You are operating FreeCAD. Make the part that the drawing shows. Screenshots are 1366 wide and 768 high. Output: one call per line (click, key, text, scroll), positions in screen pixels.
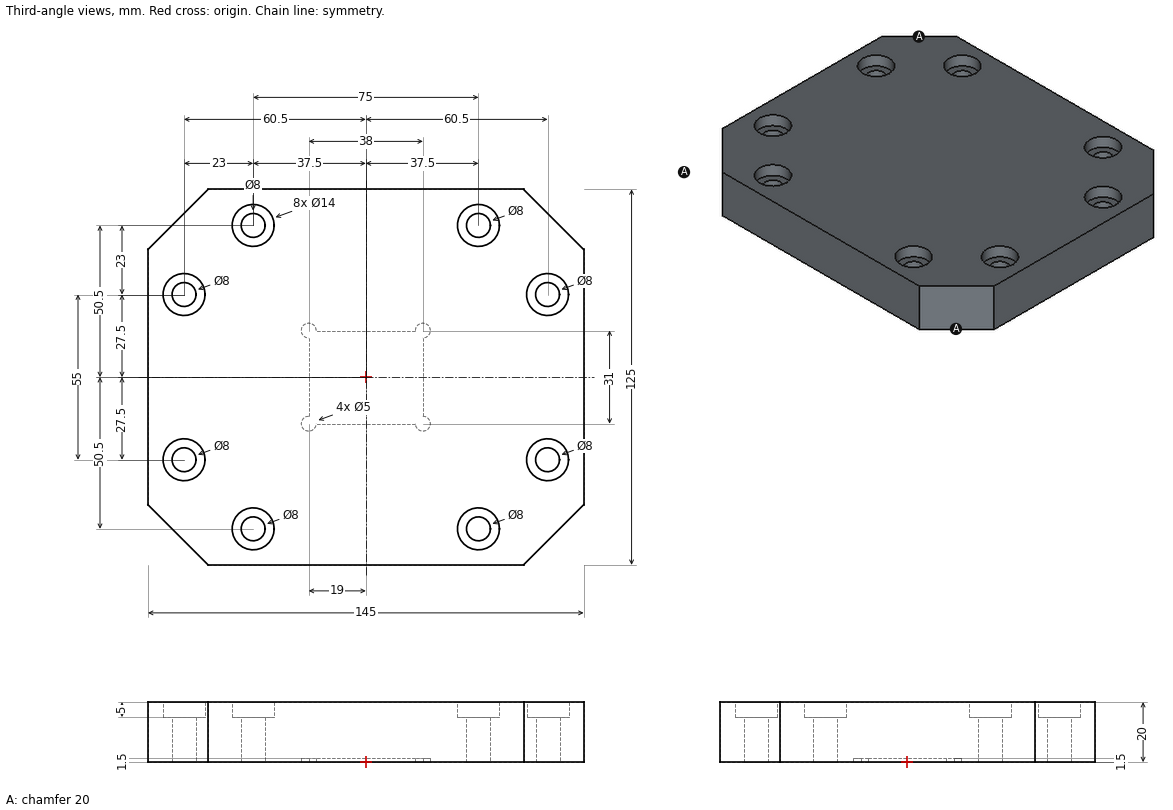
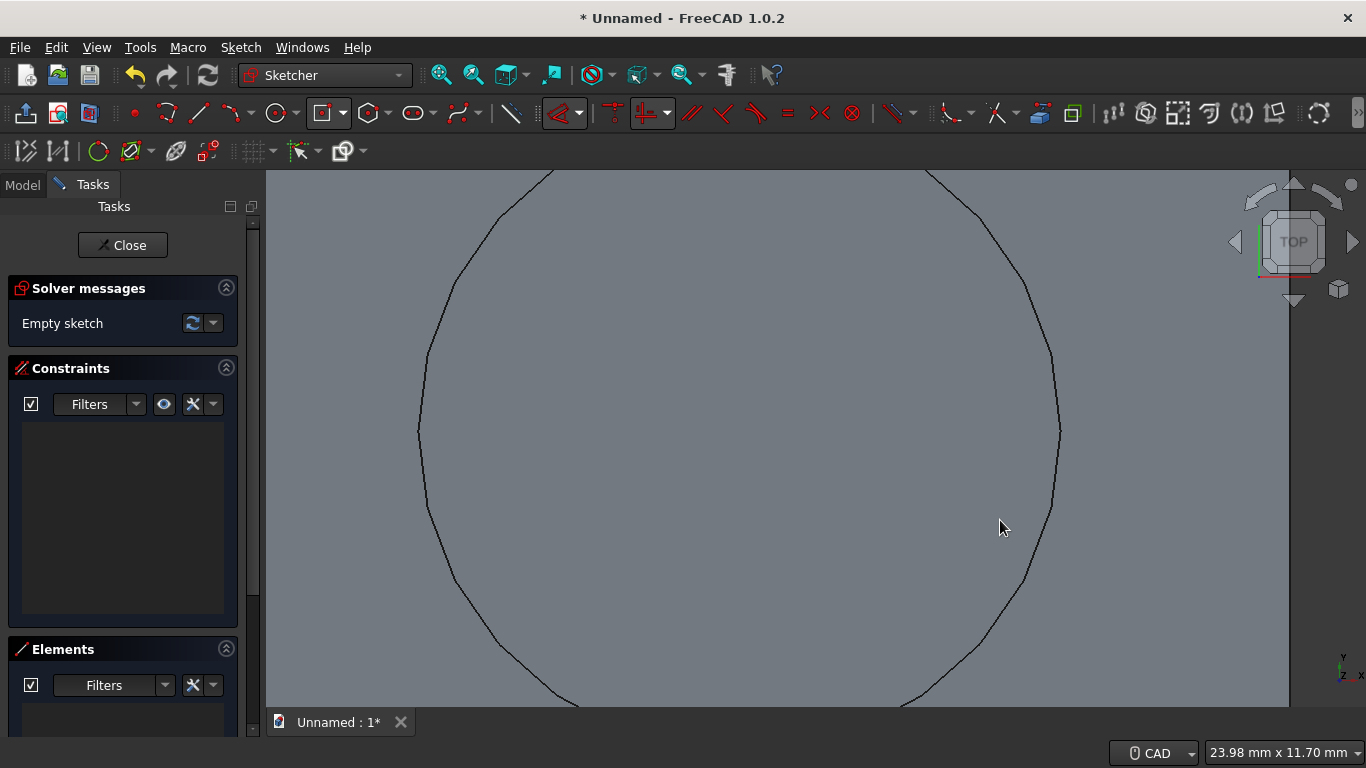
key(g)
key(c)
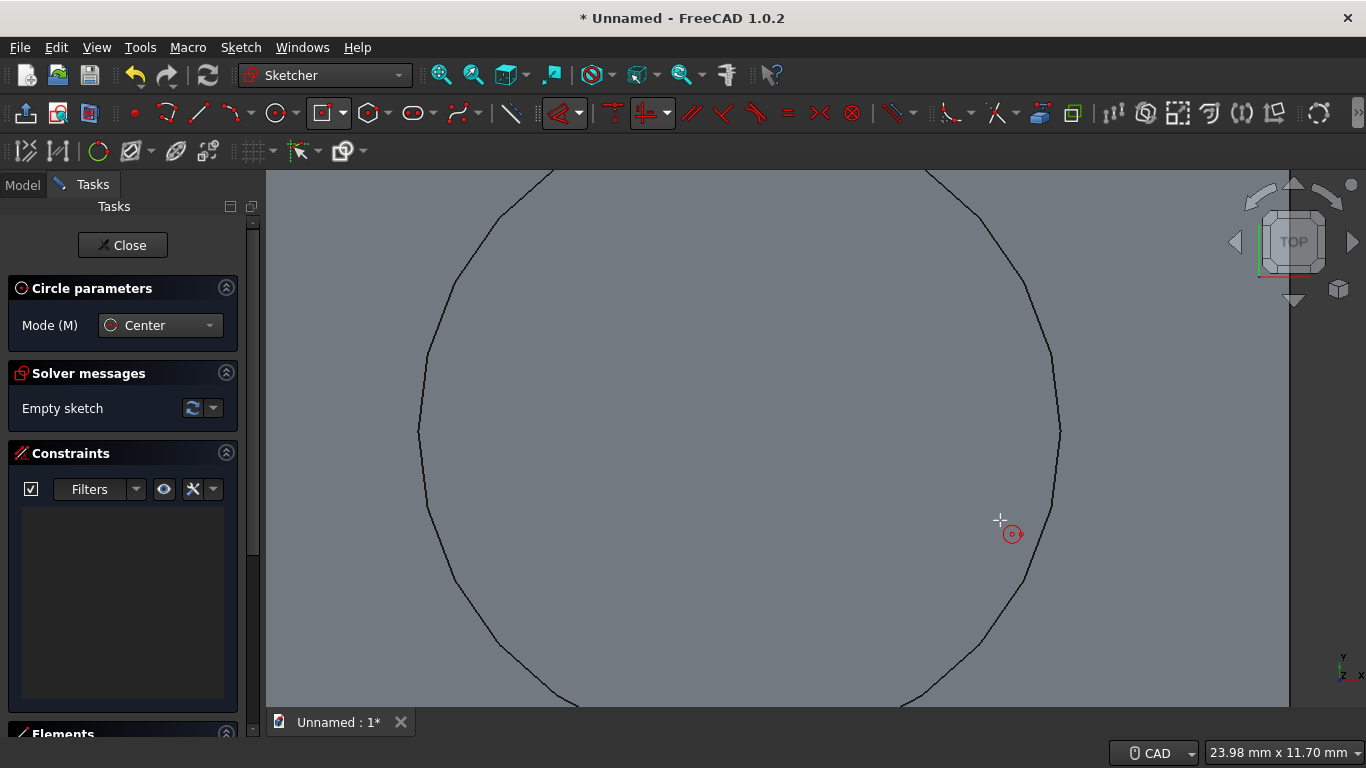
click(739, 431)
click(869, 302)
key(Escape)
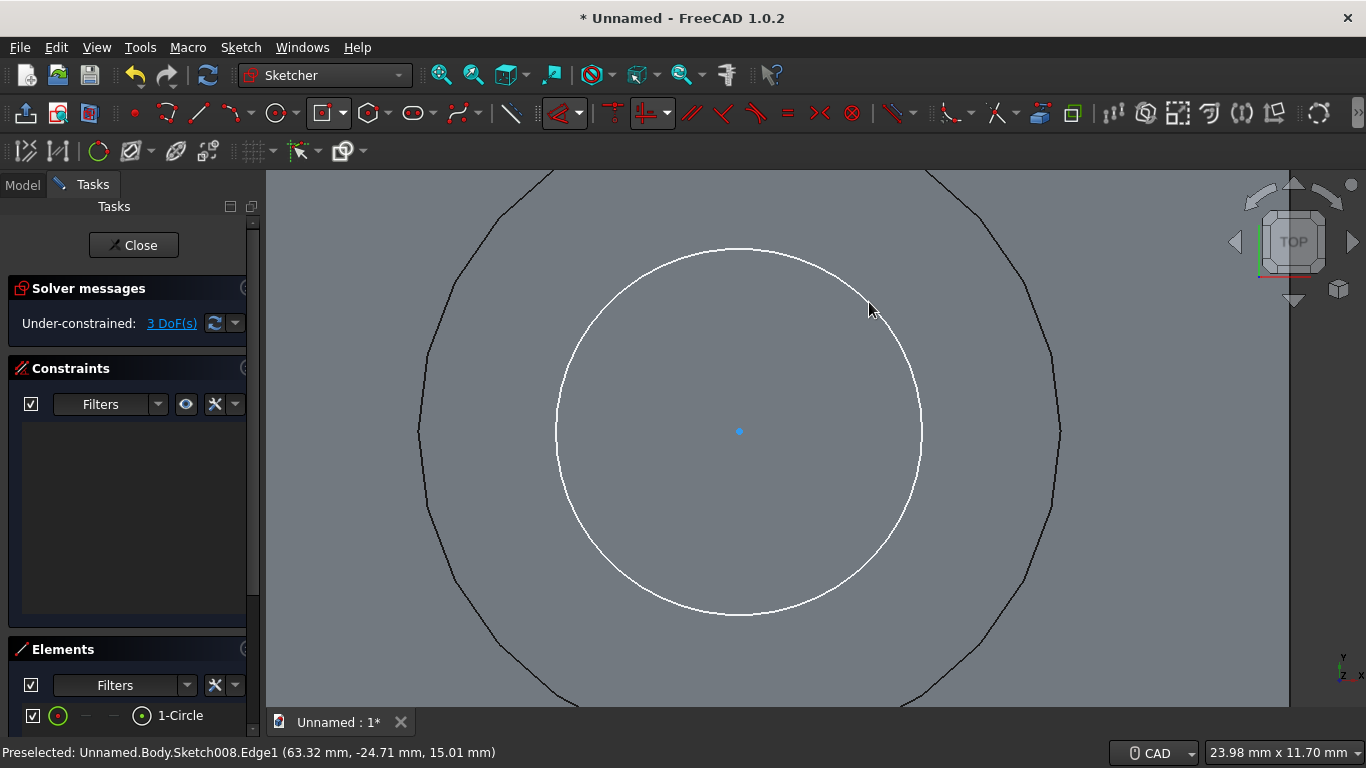
click(868, 302)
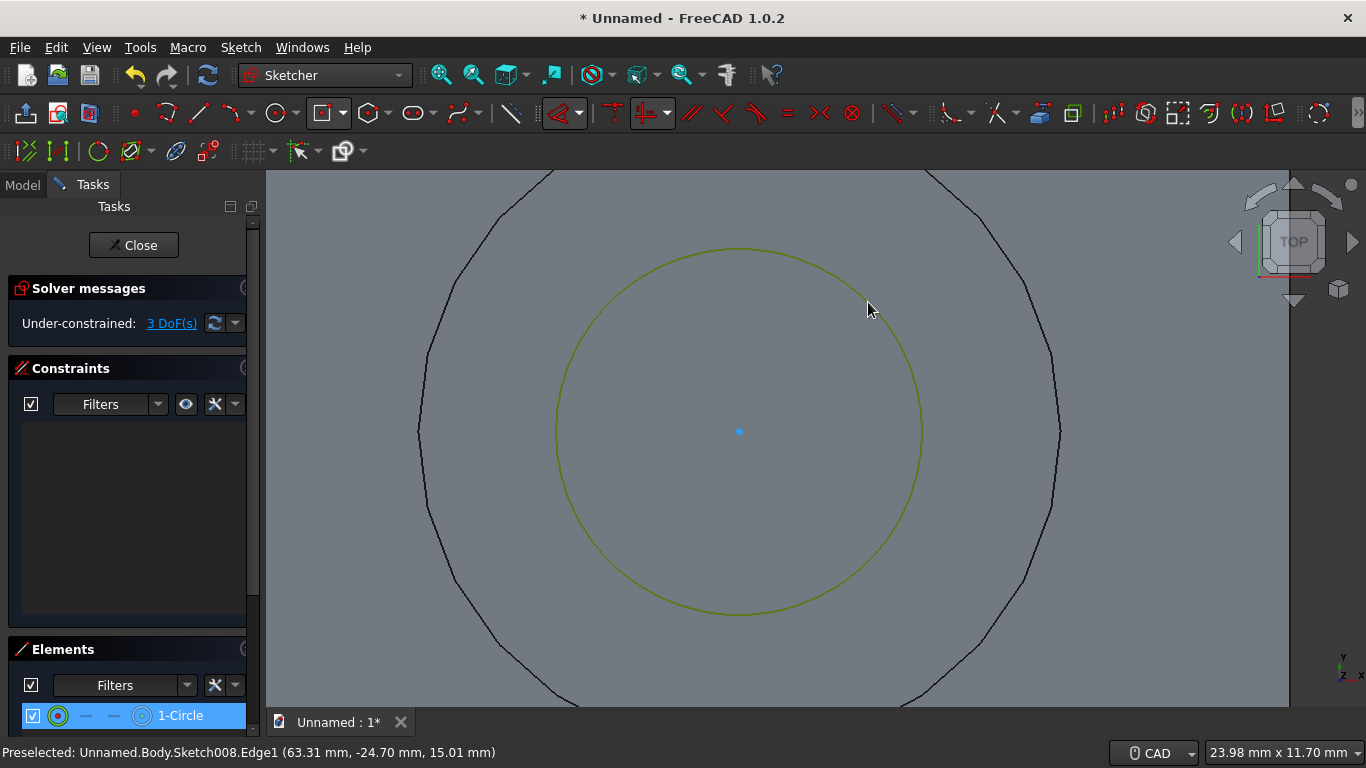
key(k)
key(o)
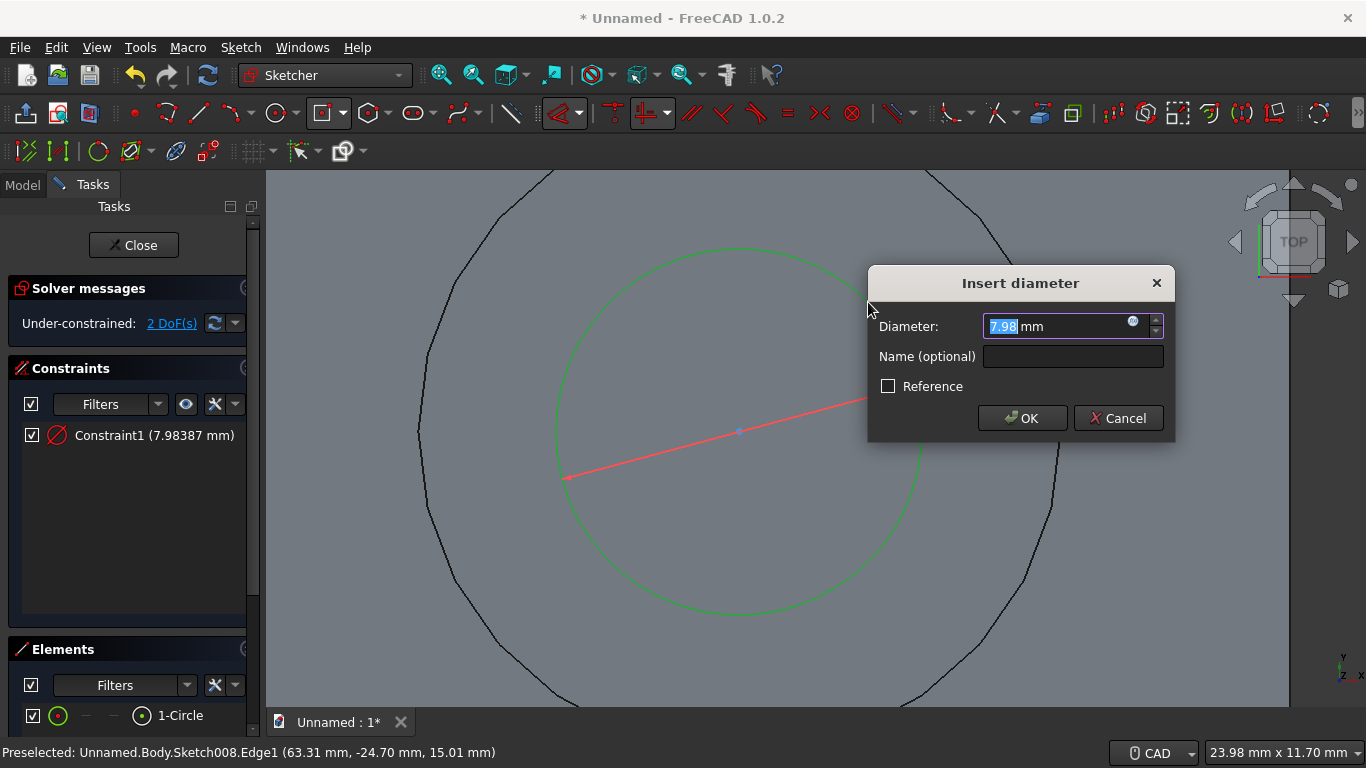
text(8)
key(Return)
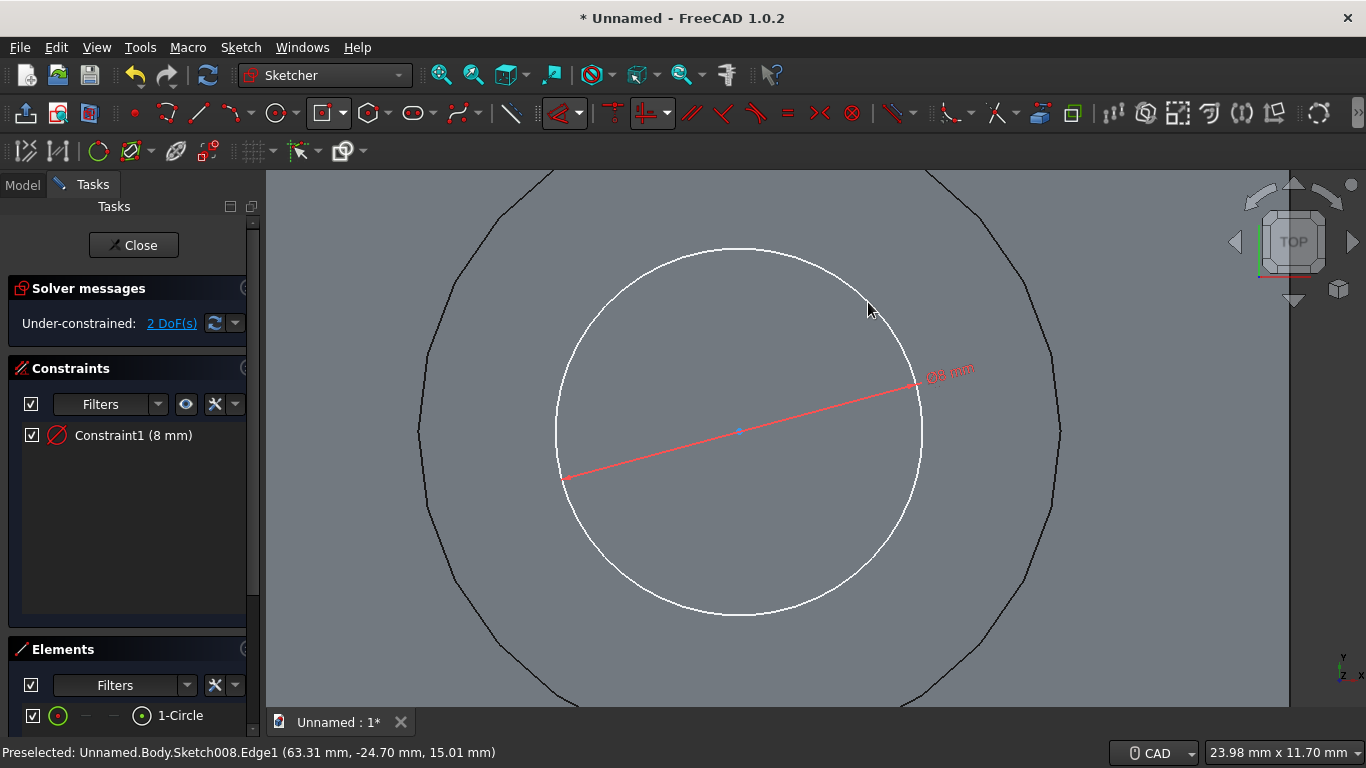
click(739, 432)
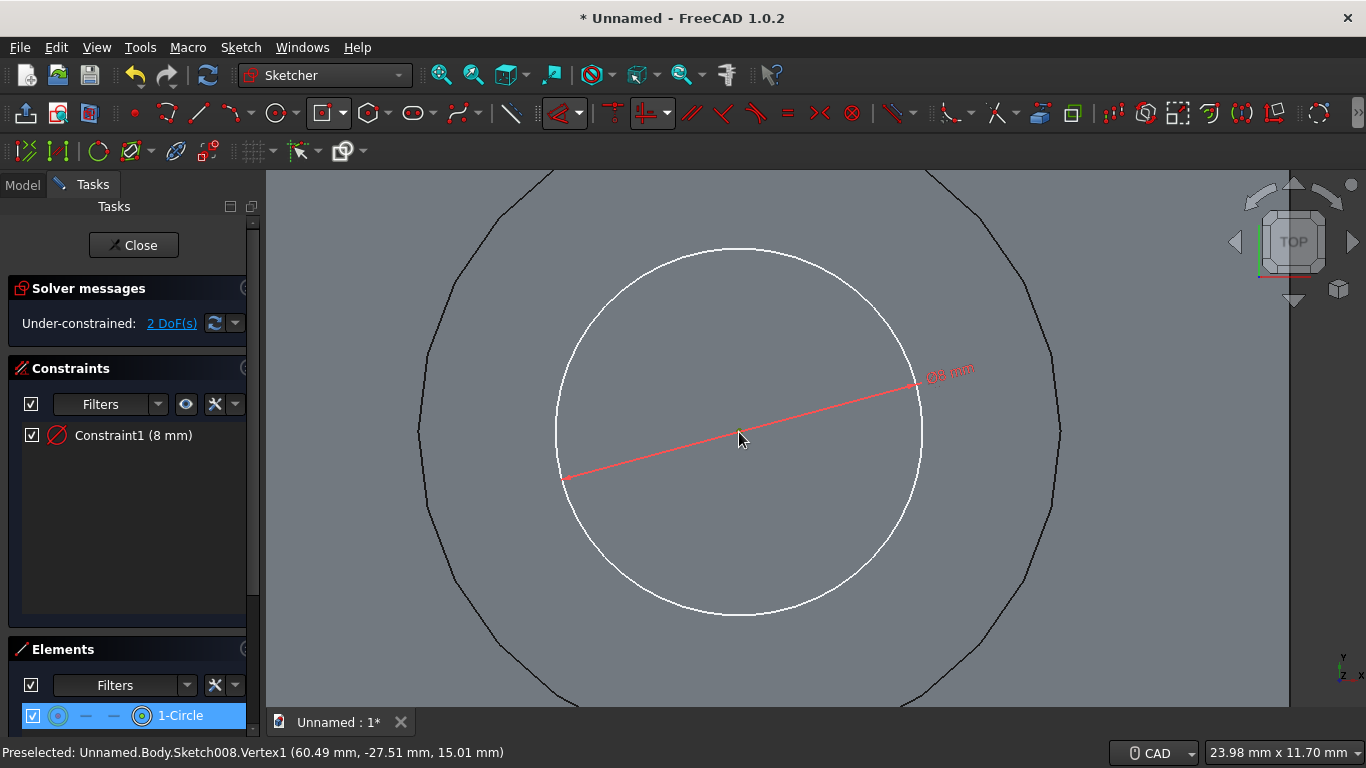
key(l)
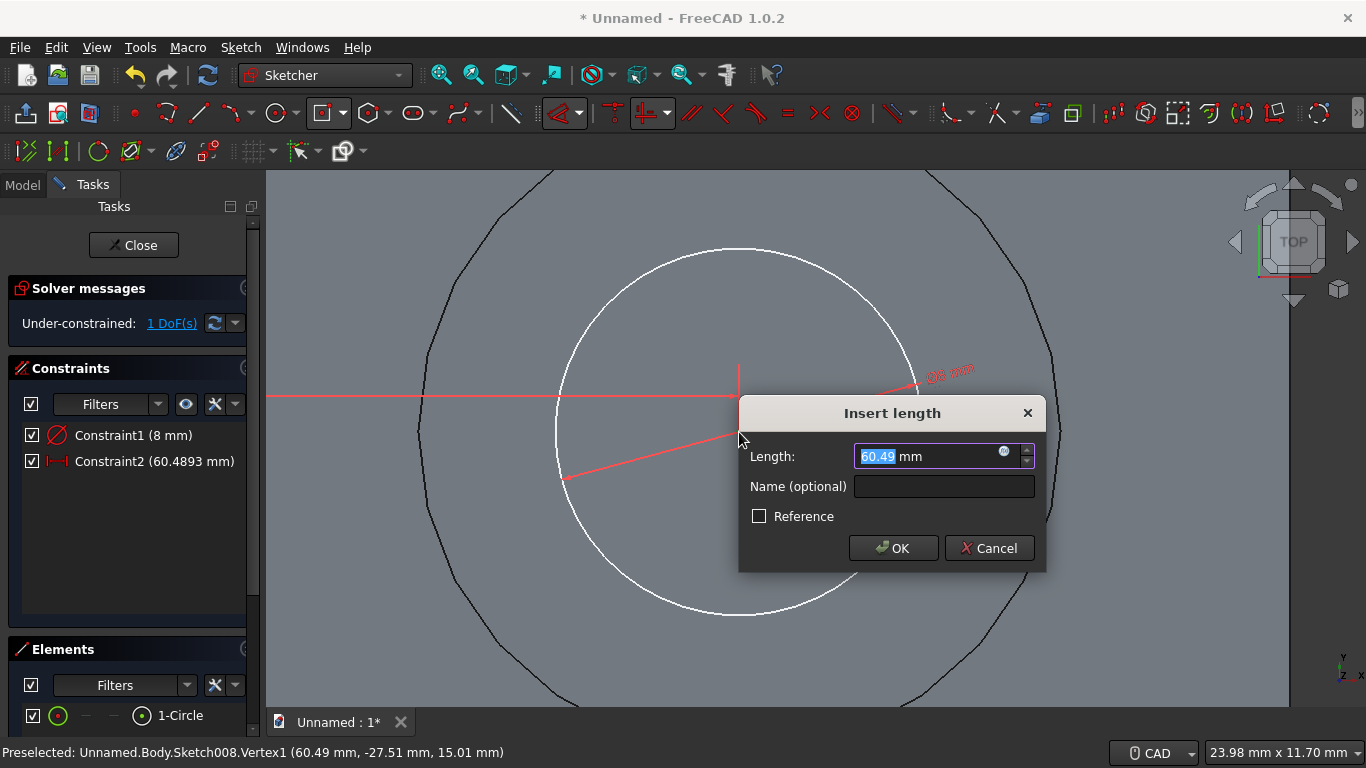
text(60.5)
key(Return)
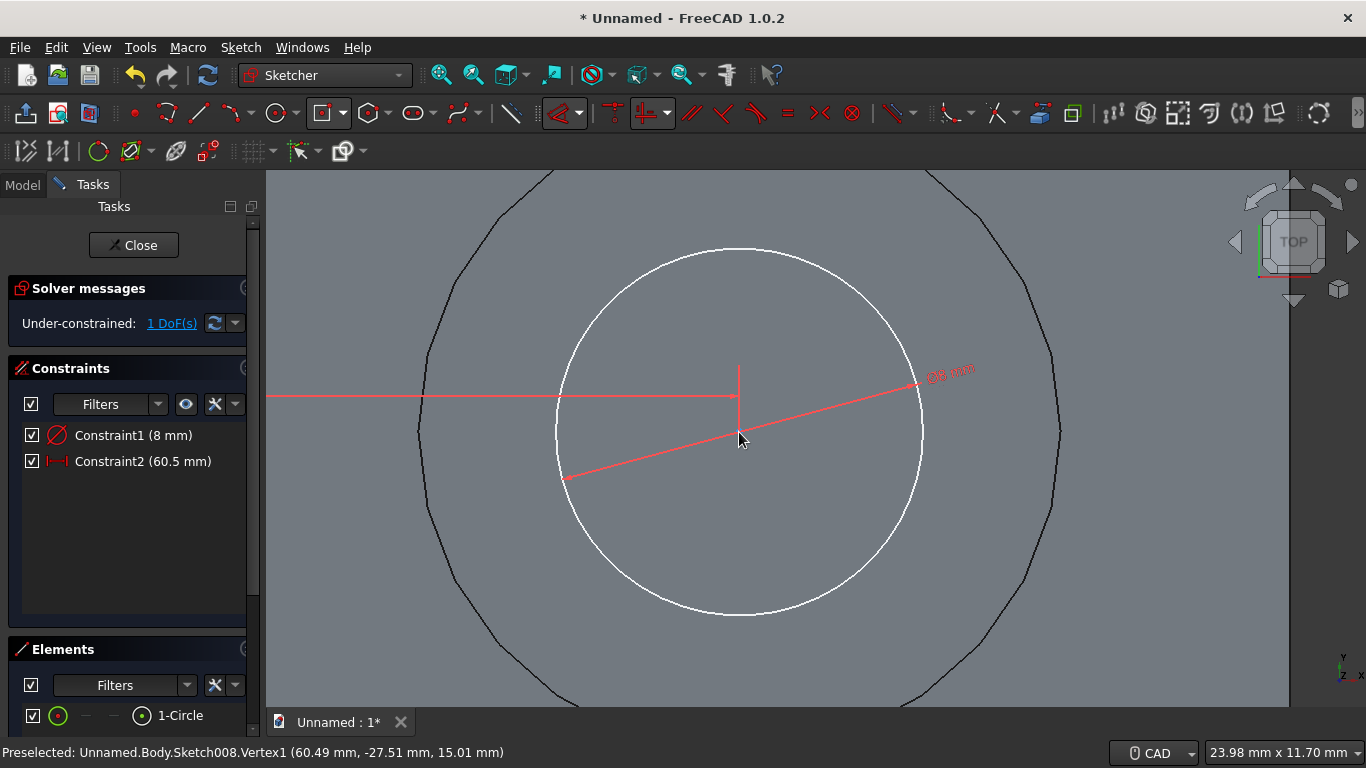
click(739, 432)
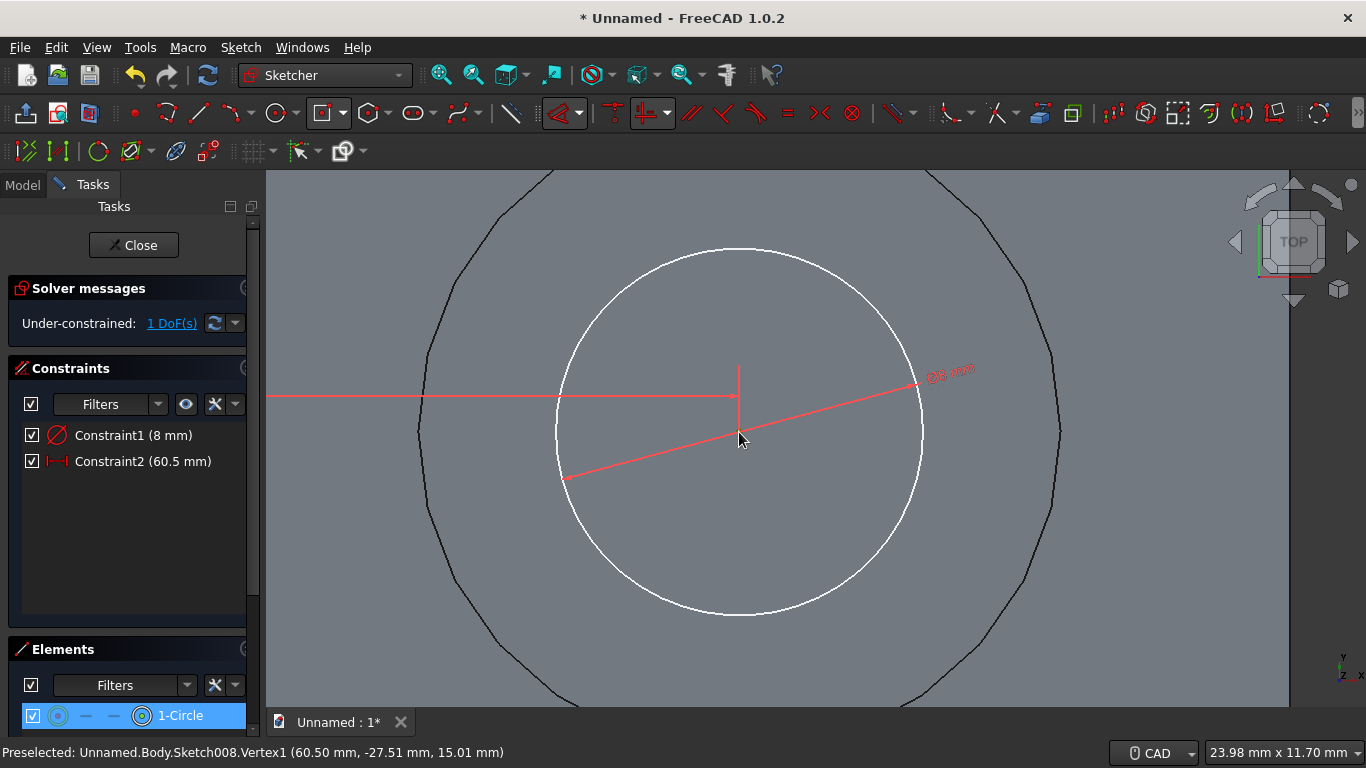
key(i)